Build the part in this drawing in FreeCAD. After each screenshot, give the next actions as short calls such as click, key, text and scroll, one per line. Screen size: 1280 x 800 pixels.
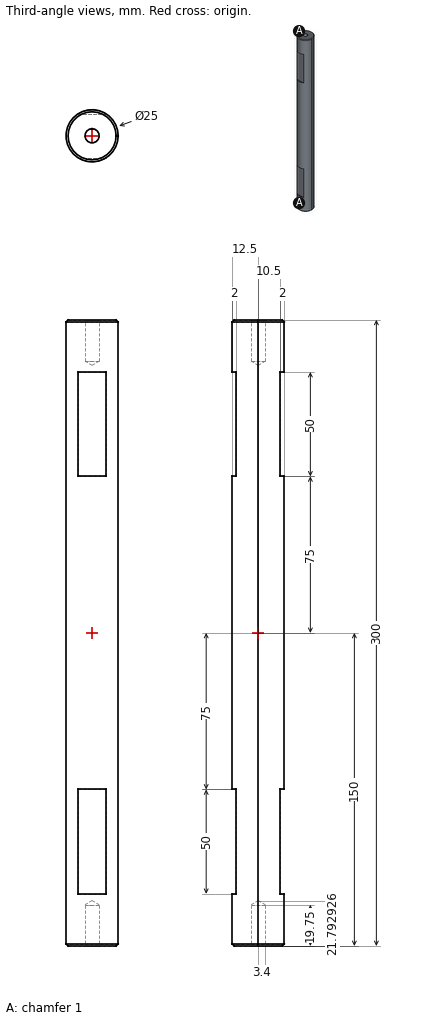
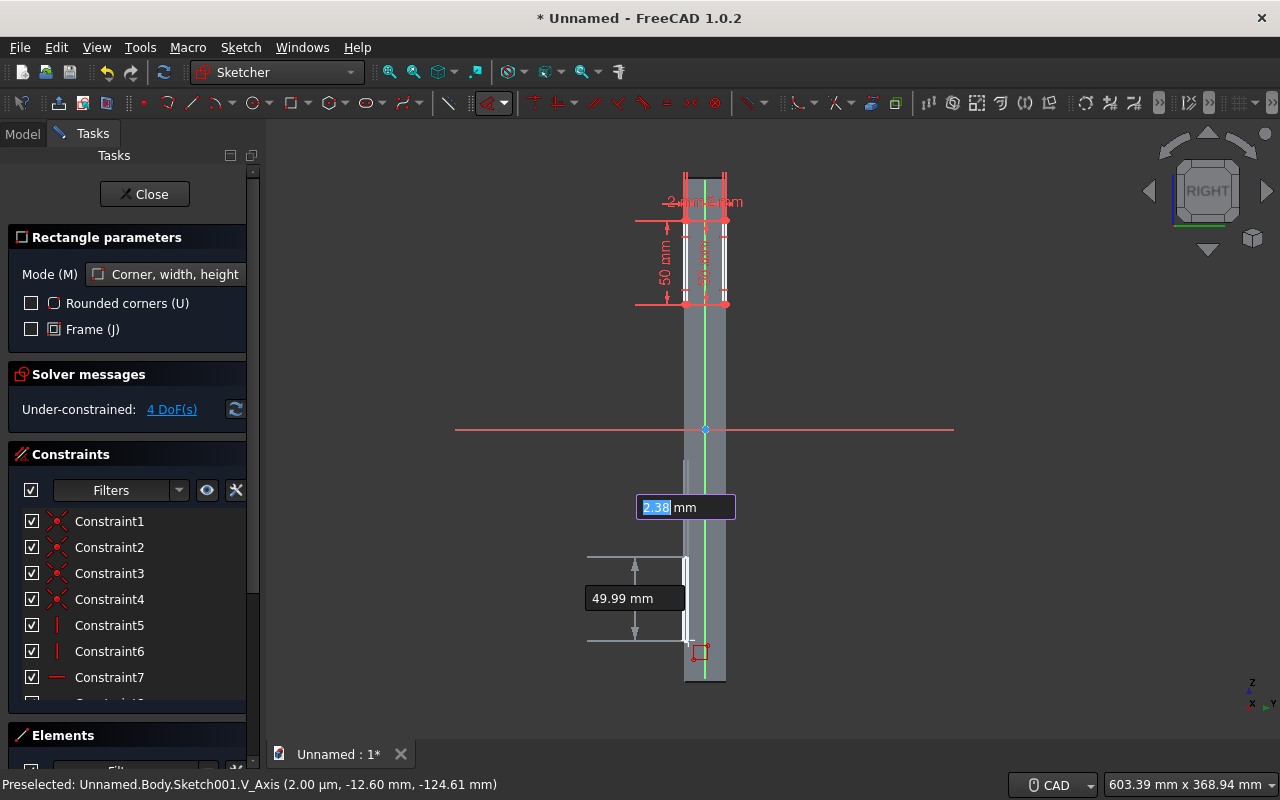
text(2)
key(Tab)
text(50)
key(Return)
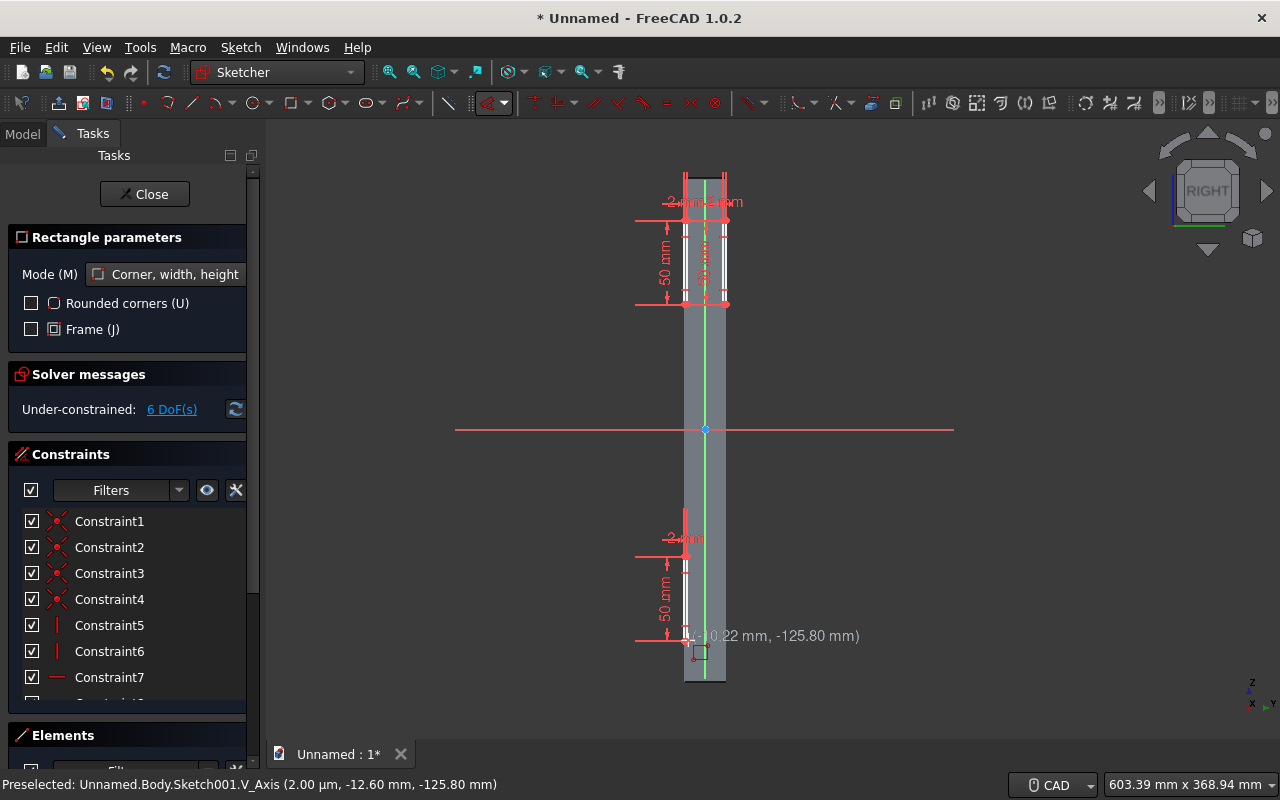
scroll(723, 556, up, 8)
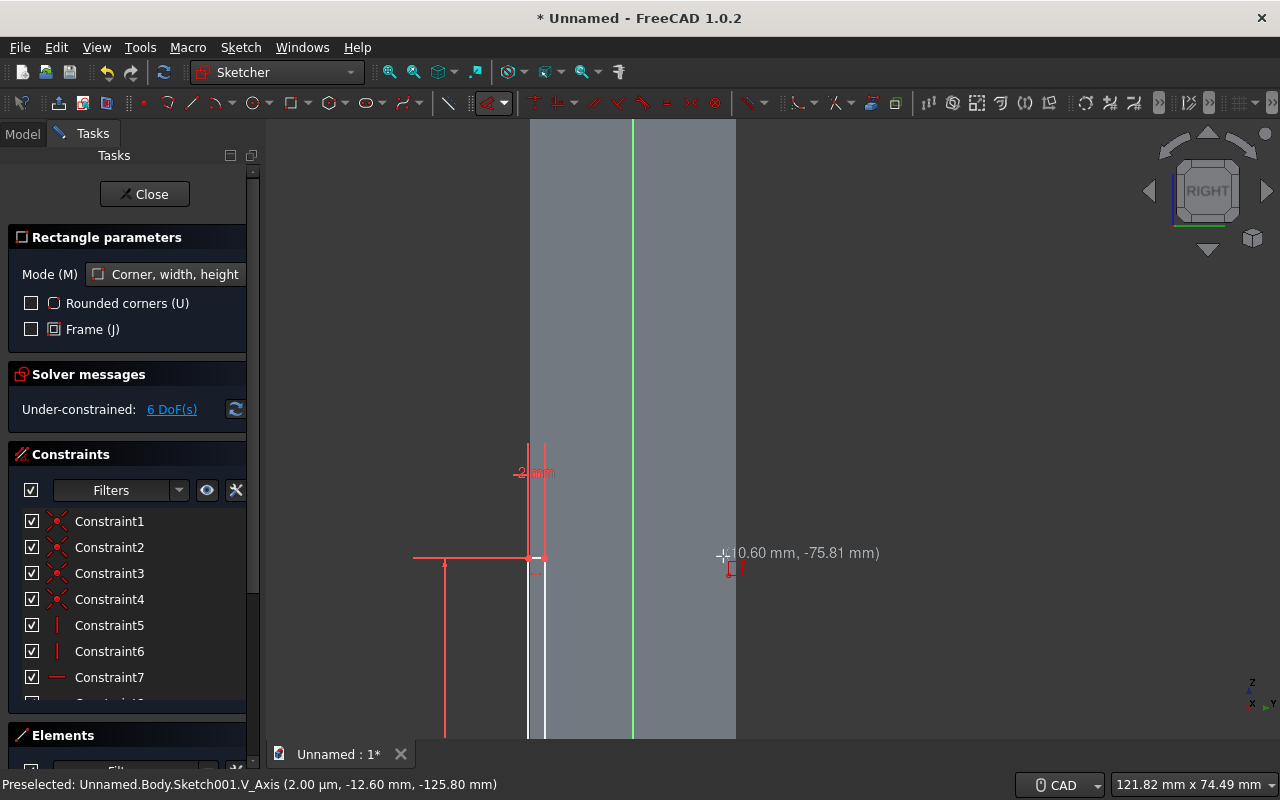
scroll(723, 556, down, 8)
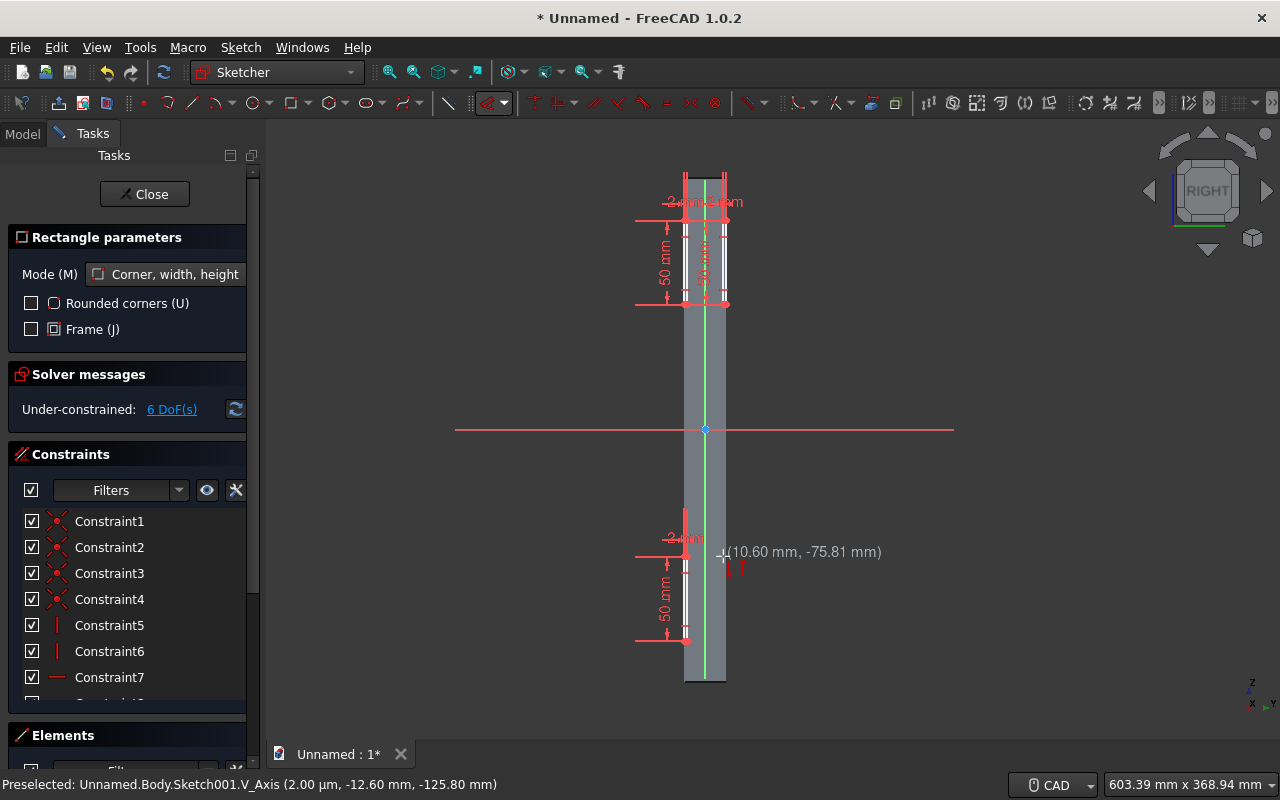
click(723, 556)
move(726, 640)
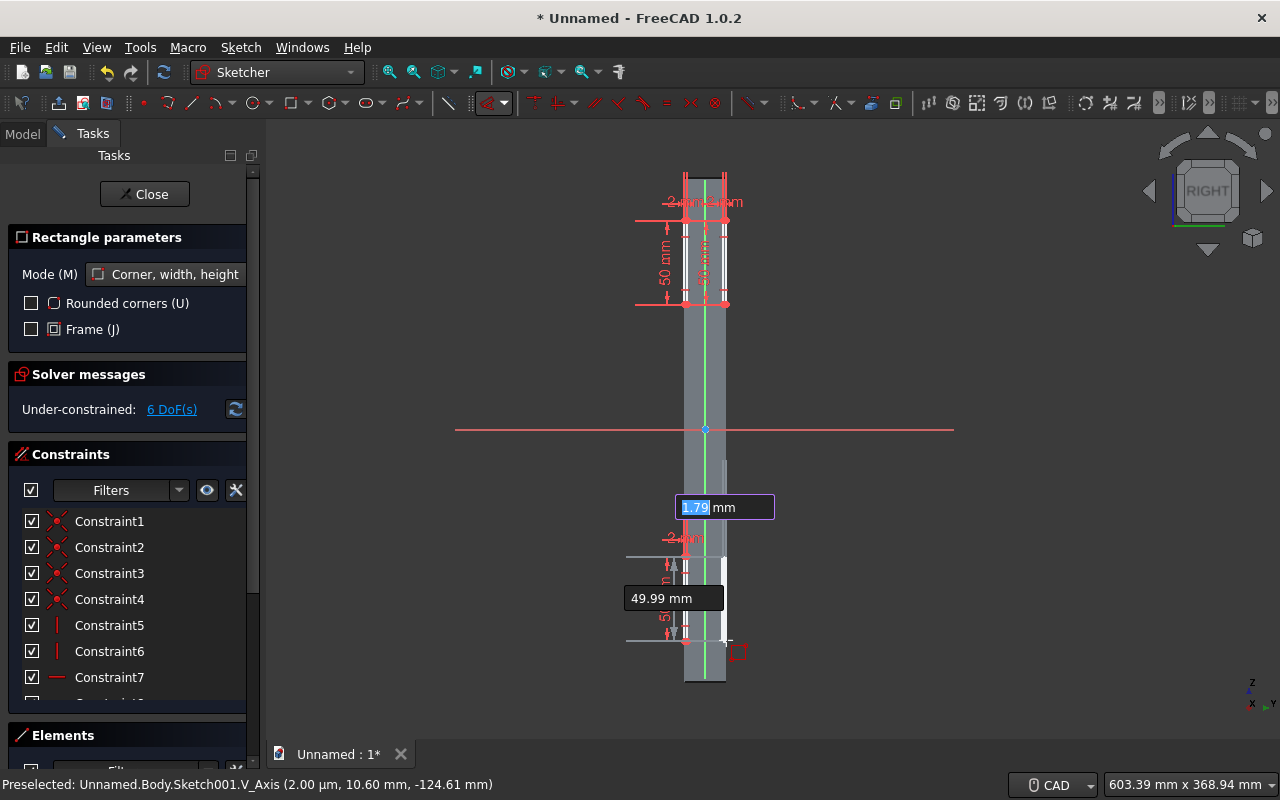
text(2)
key(Tab)
text(50)
key(Return)
key(Escape)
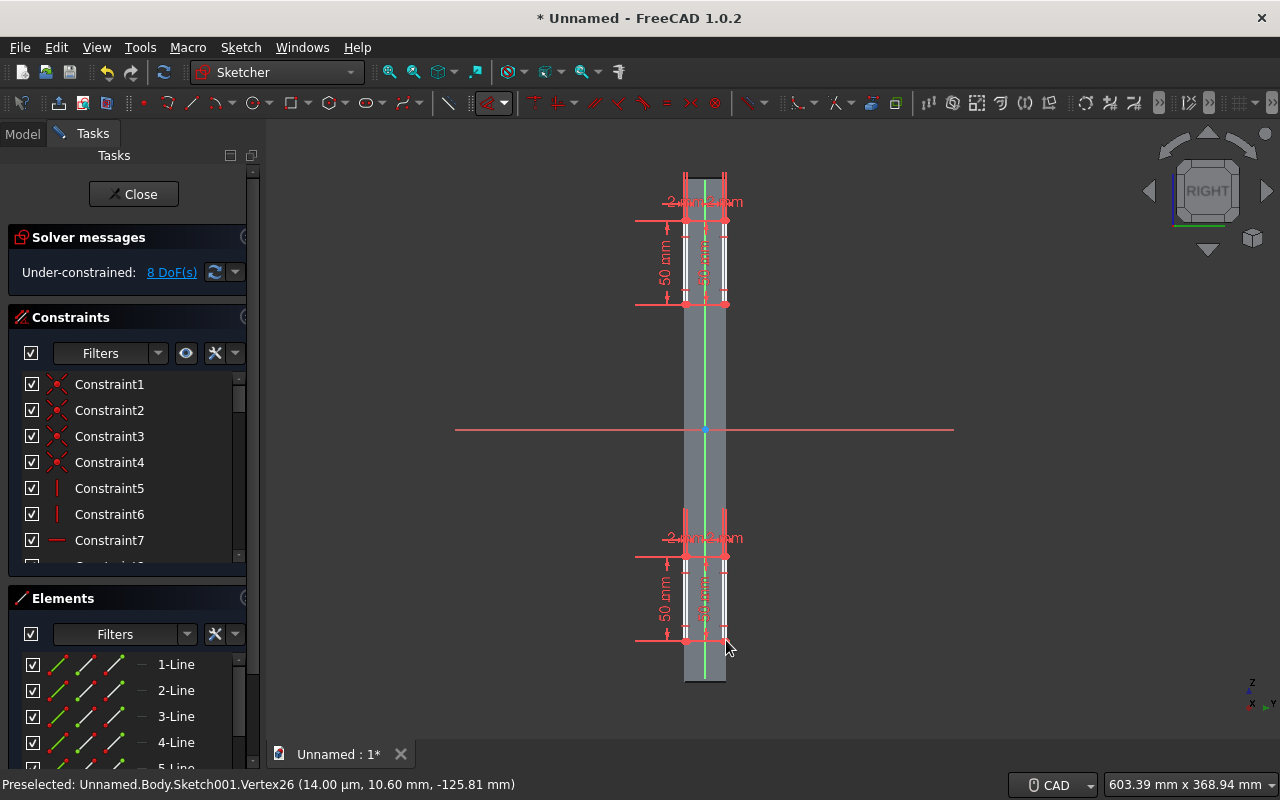
click(488, 104)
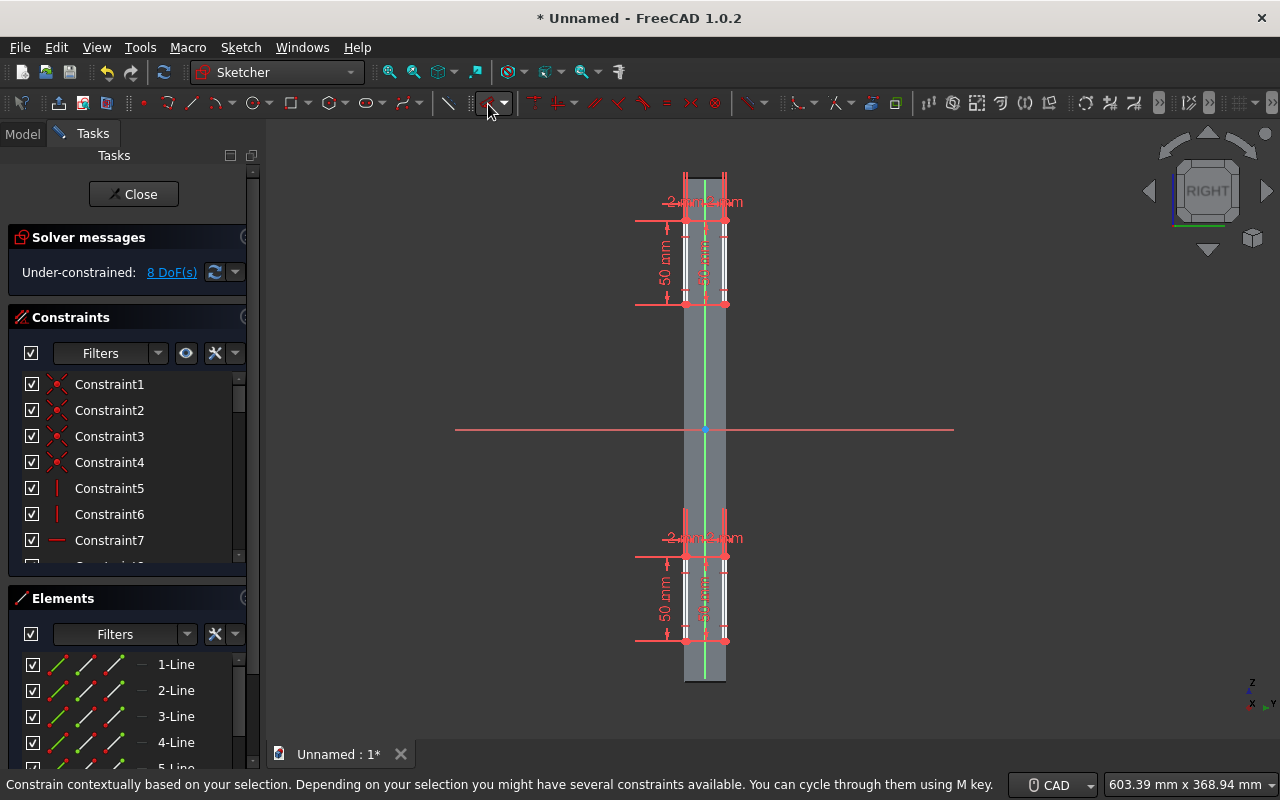
scroll(723, 305, up, 7)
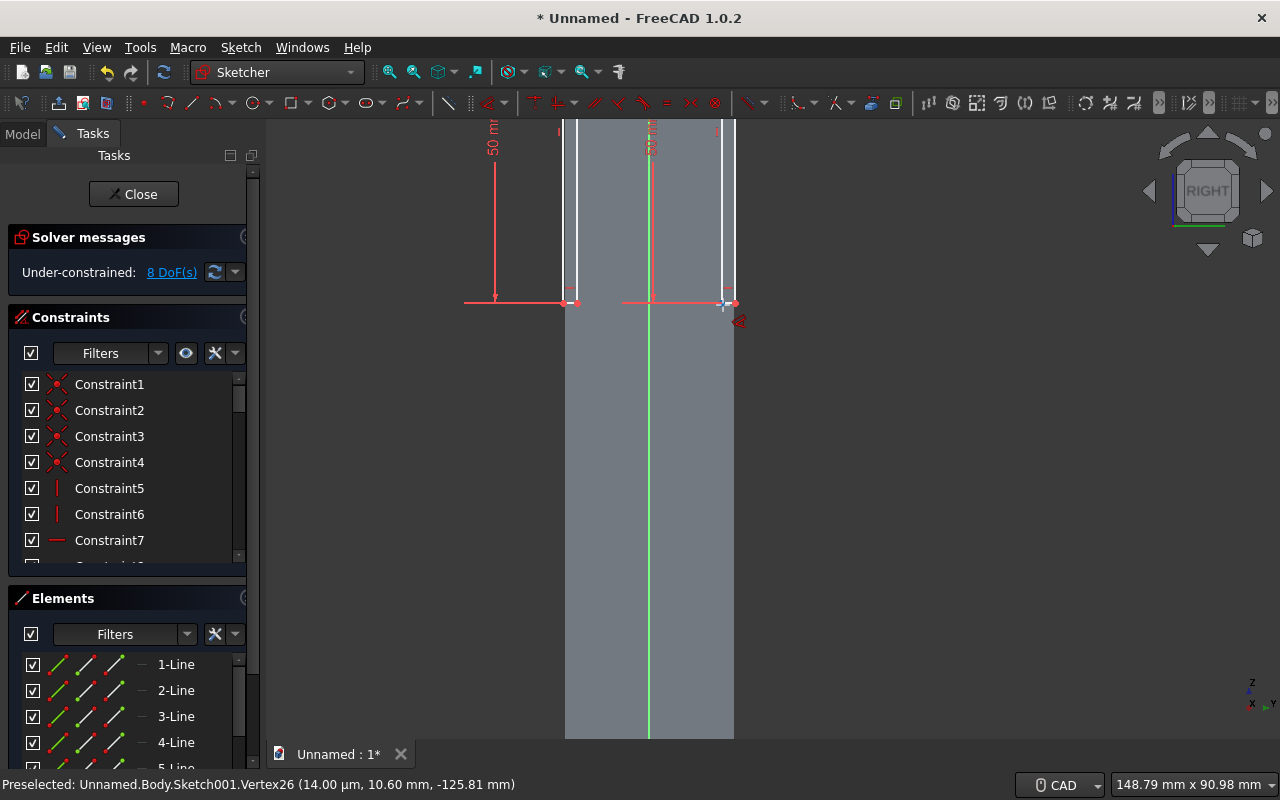
click(722, 303)
click(756, 507)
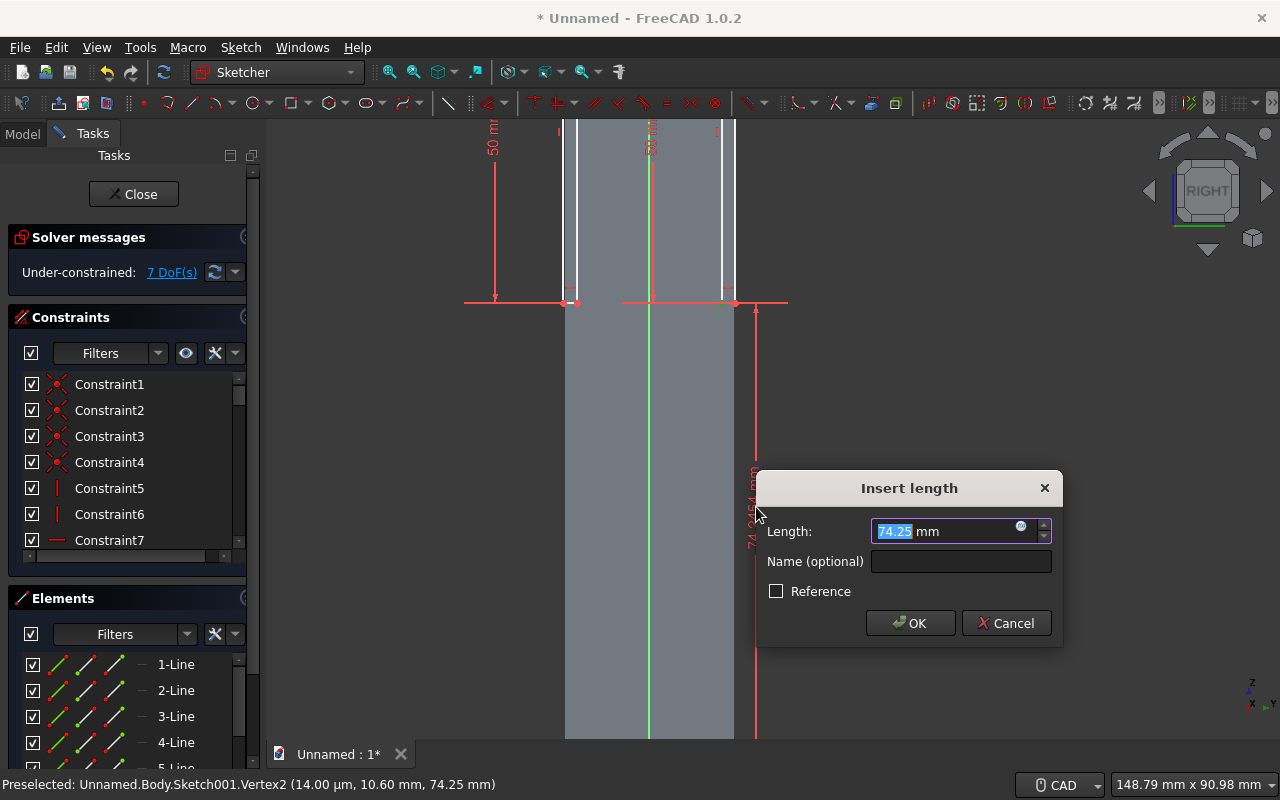
text(75)
key(Return)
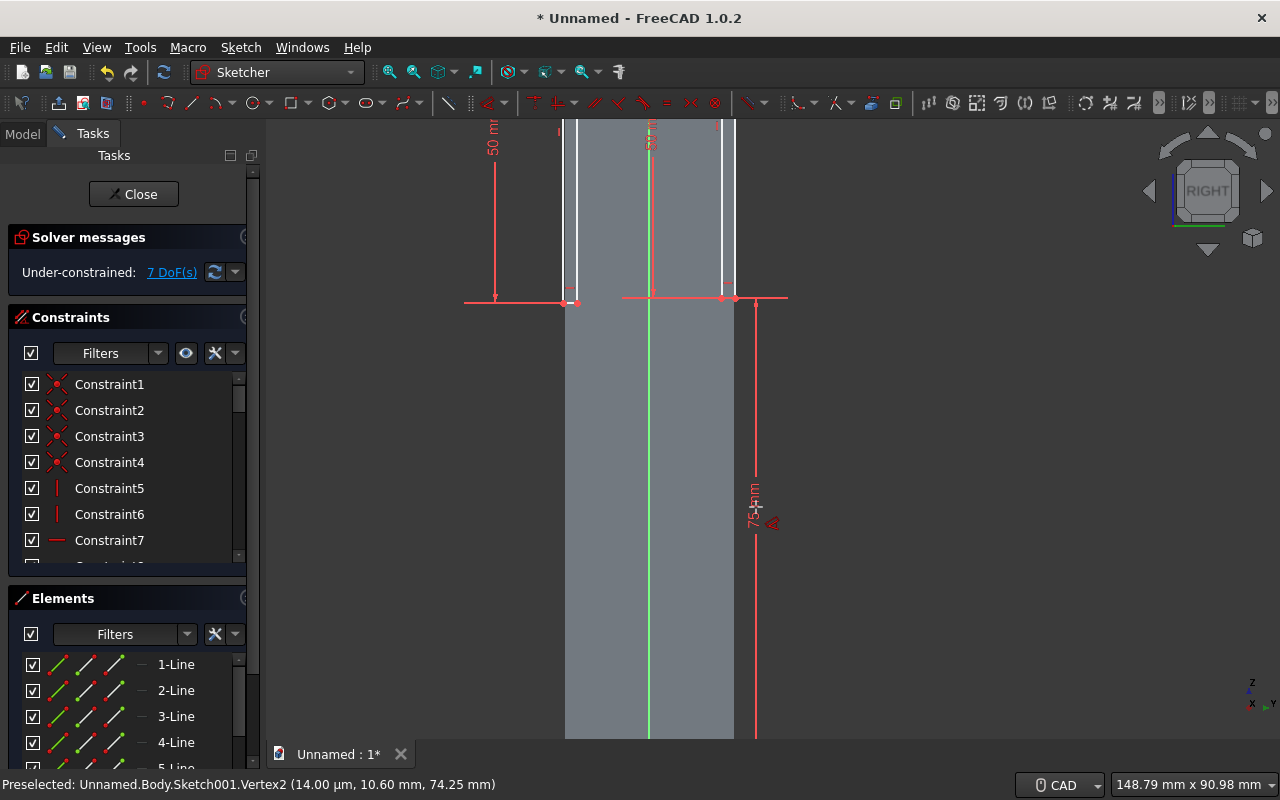
click(563, 303)
click(529, 507)